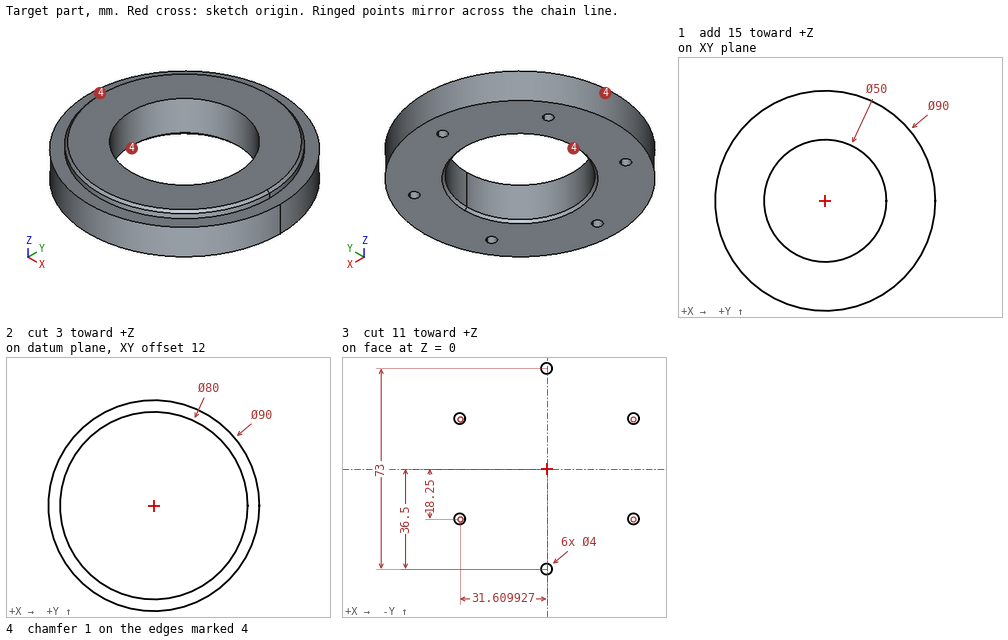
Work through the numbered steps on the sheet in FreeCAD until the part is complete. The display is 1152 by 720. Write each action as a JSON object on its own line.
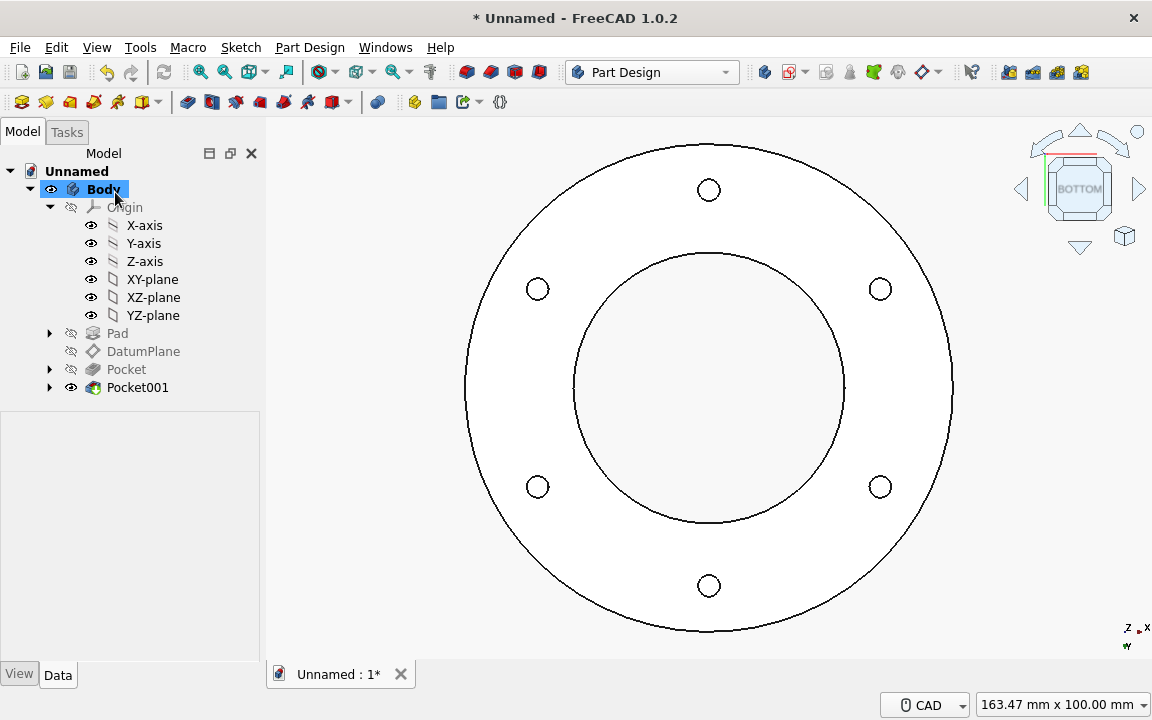
{"action": "left_click", "coordinate": [599, 307]}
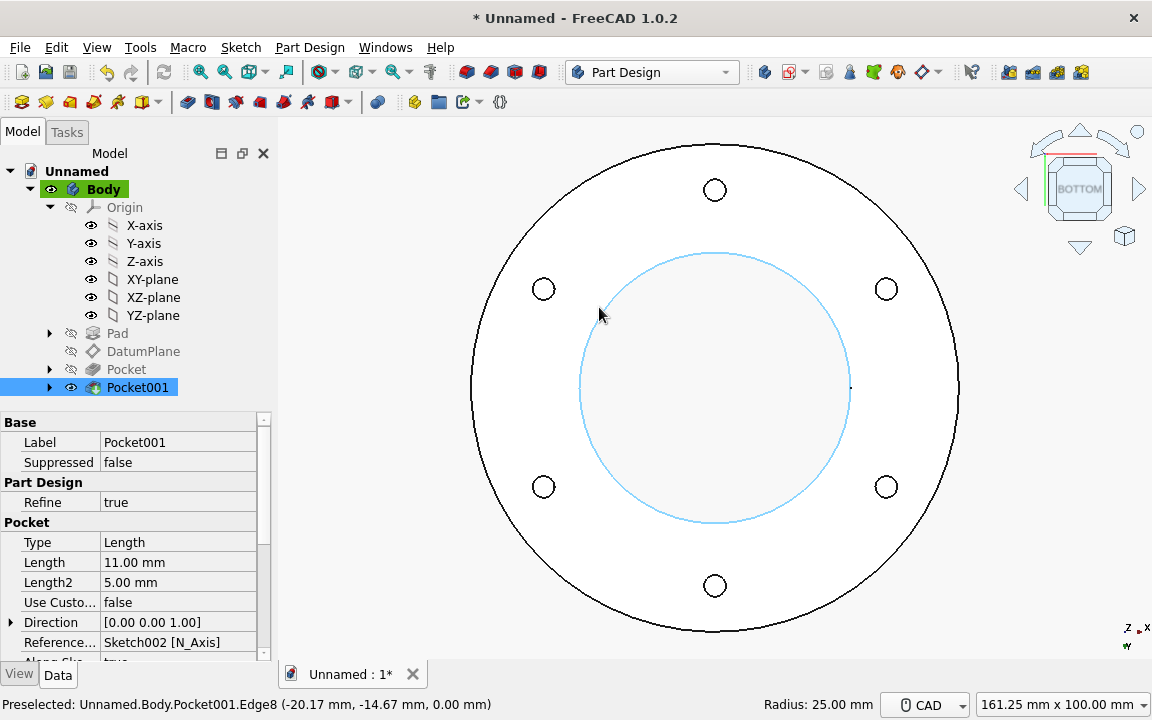
{"action": "key", "text": "0"}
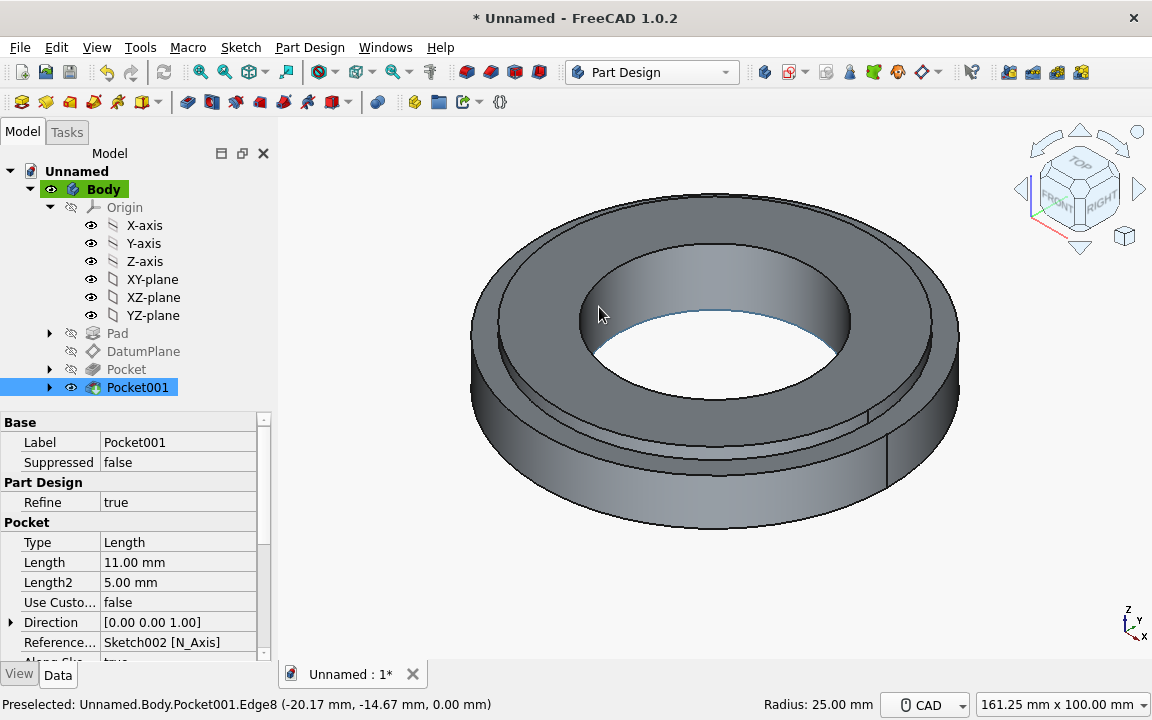
{"action": "left_click", "coordinate": [522, 377], "text": "ctrl"}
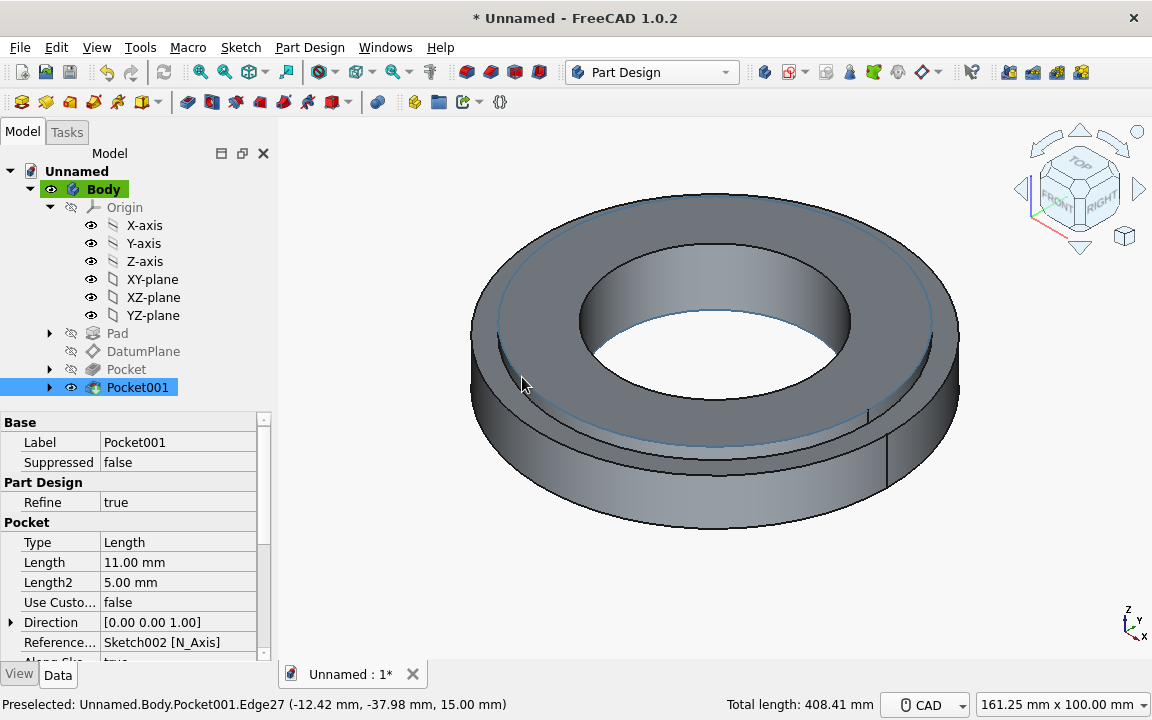
{"action": "left_click", "coordinate": [492, 72]}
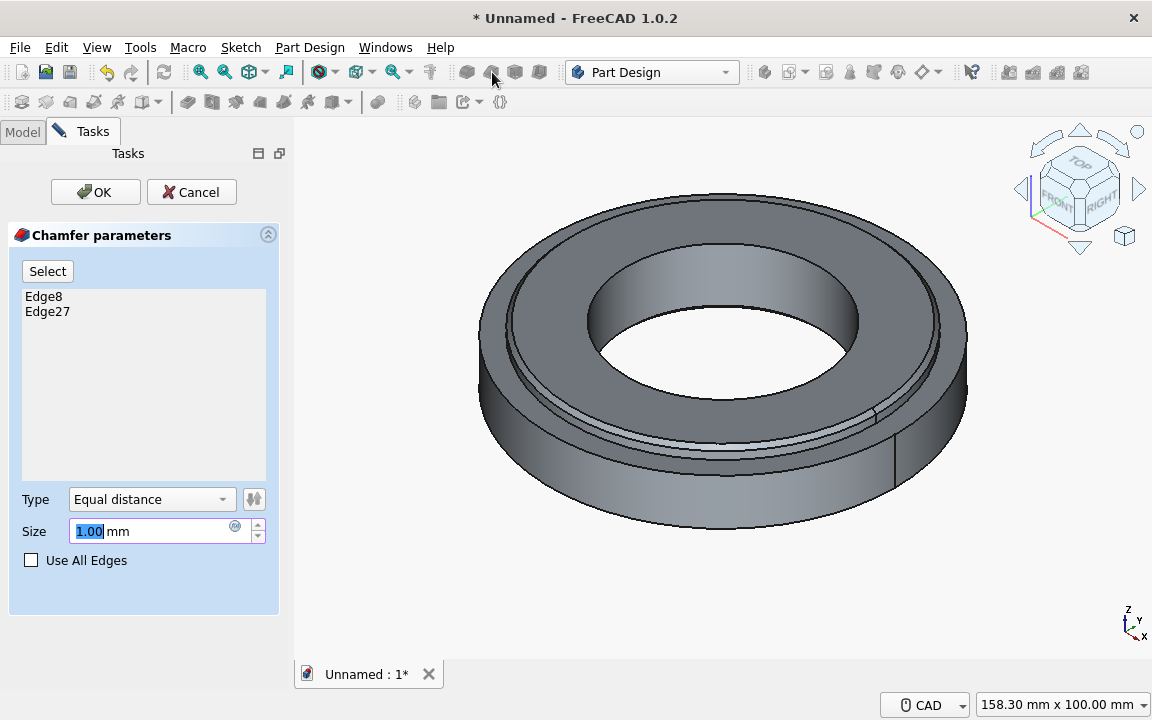
{"action": "type", "text": "1"}
{"action": "key", "text": "Tab"}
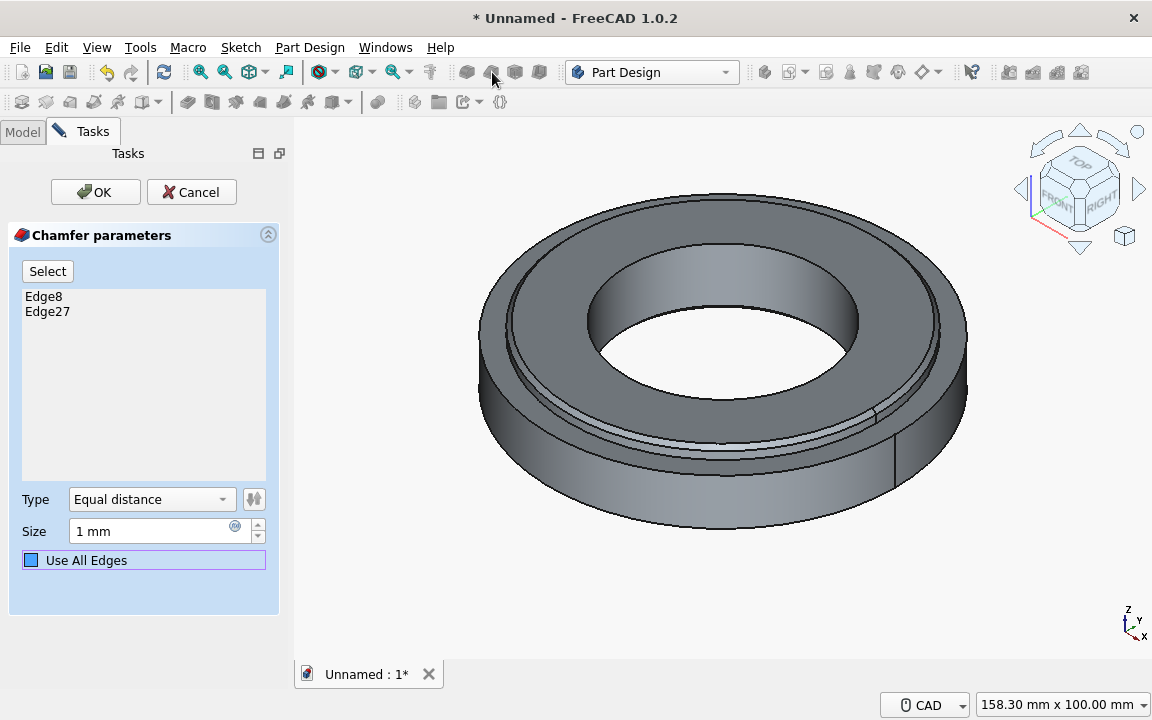
{"action": "left_click", "coordinate": [96, 192]}